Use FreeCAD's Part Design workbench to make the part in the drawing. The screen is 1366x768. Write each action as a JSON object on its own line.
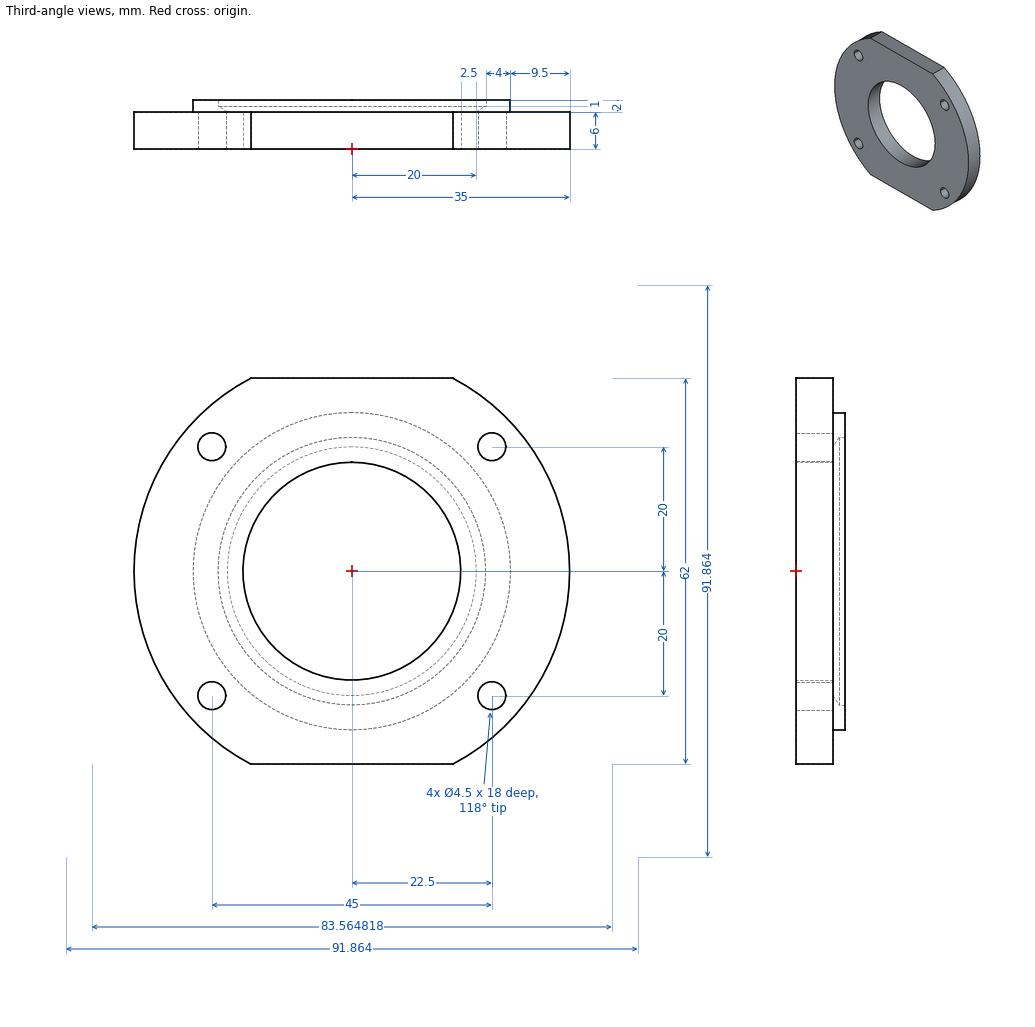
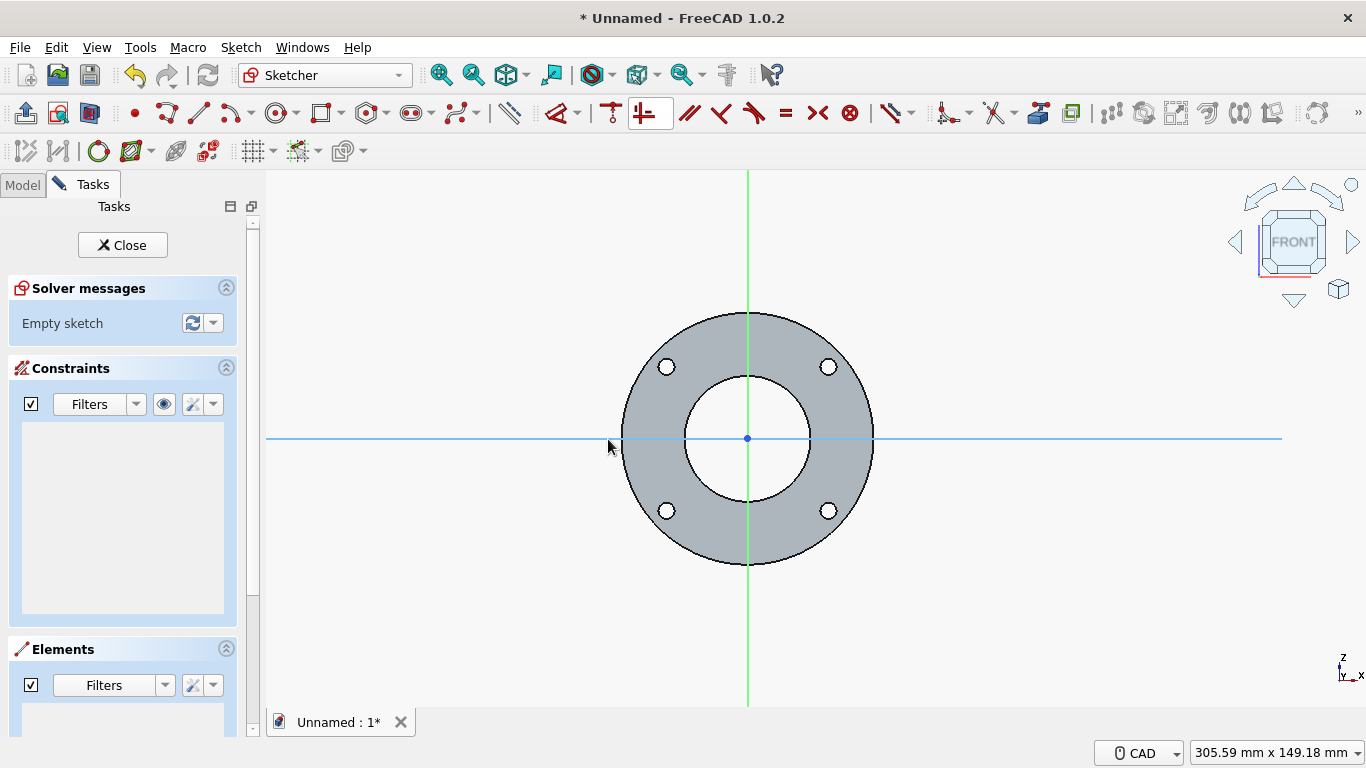
{"action": "left_click", "coordinate": [344, 114]}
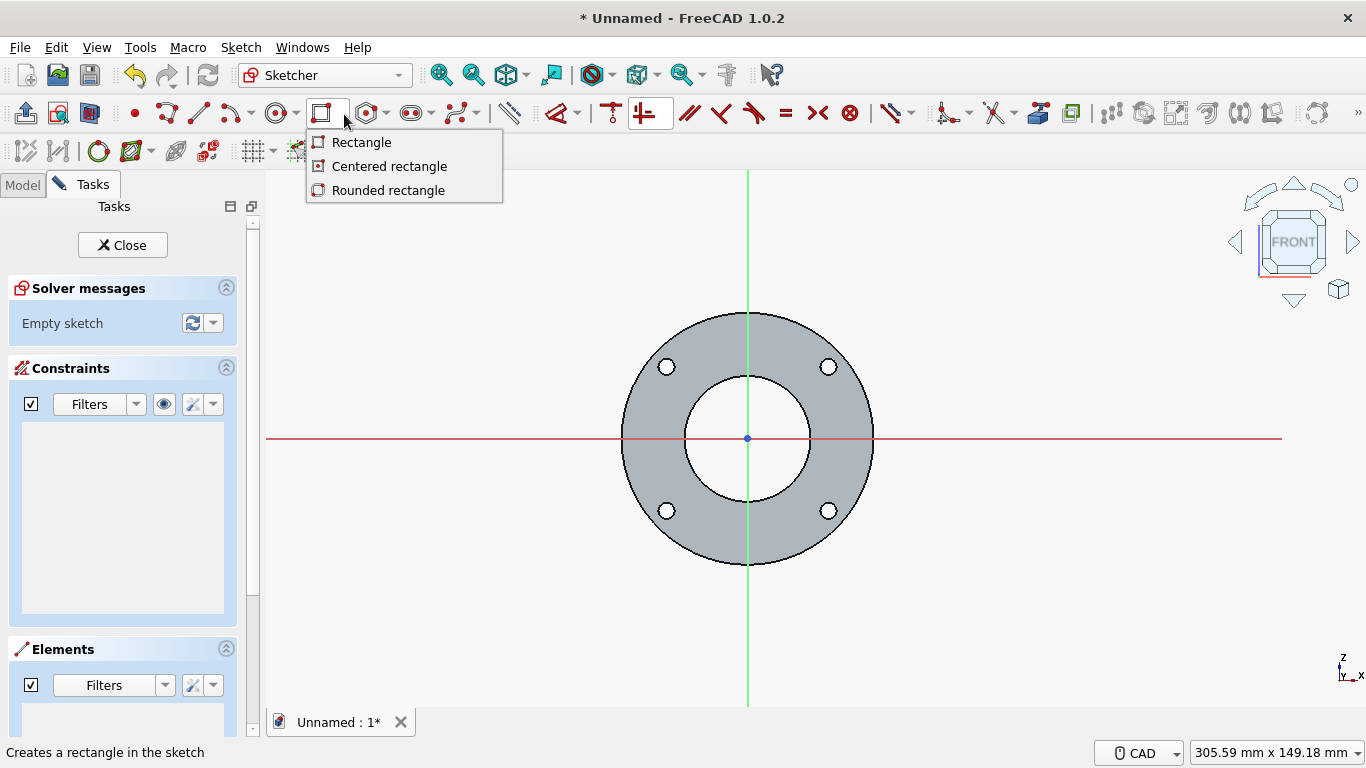
{"action": "left_click", "coordinate": [404, 166]}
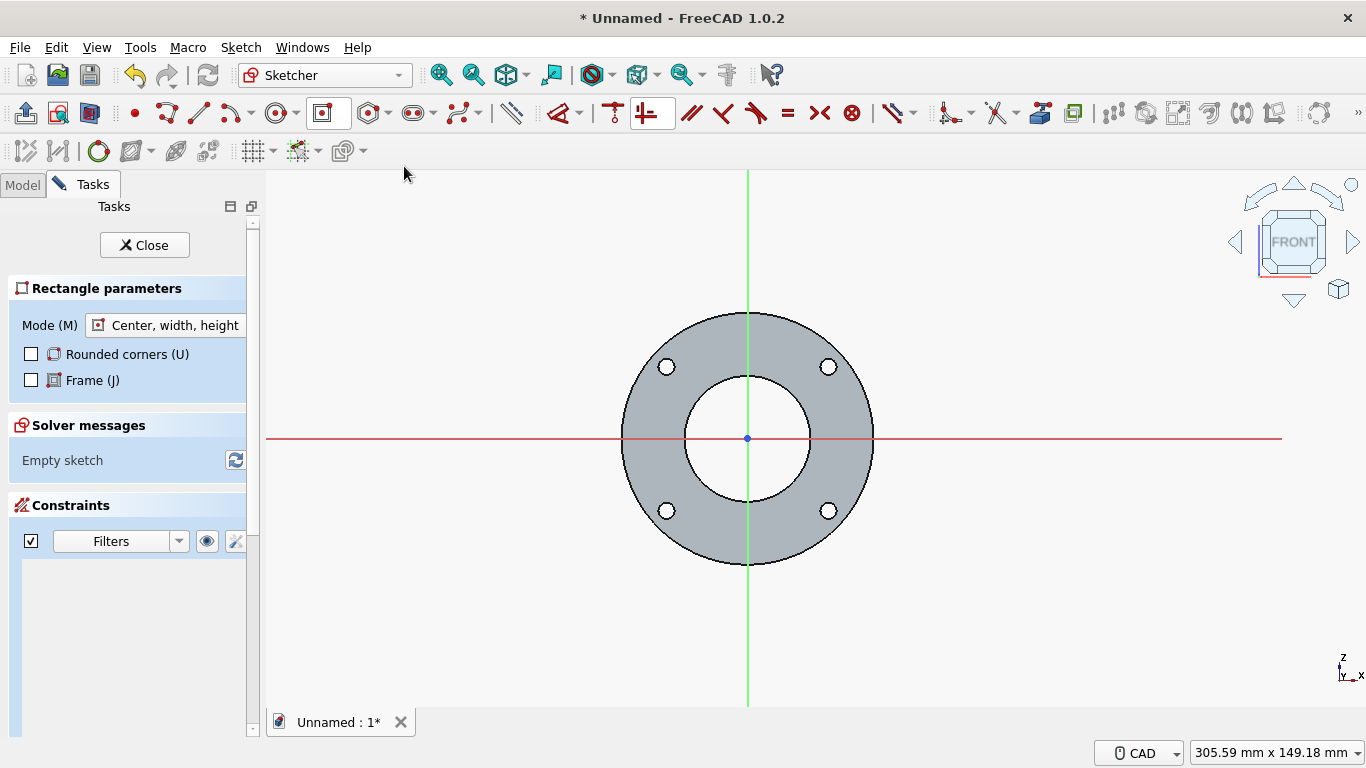
{"action": "left_click", "coordinate": [748, 439]}
{"action": "left_click", "coordinate": [913, 273]}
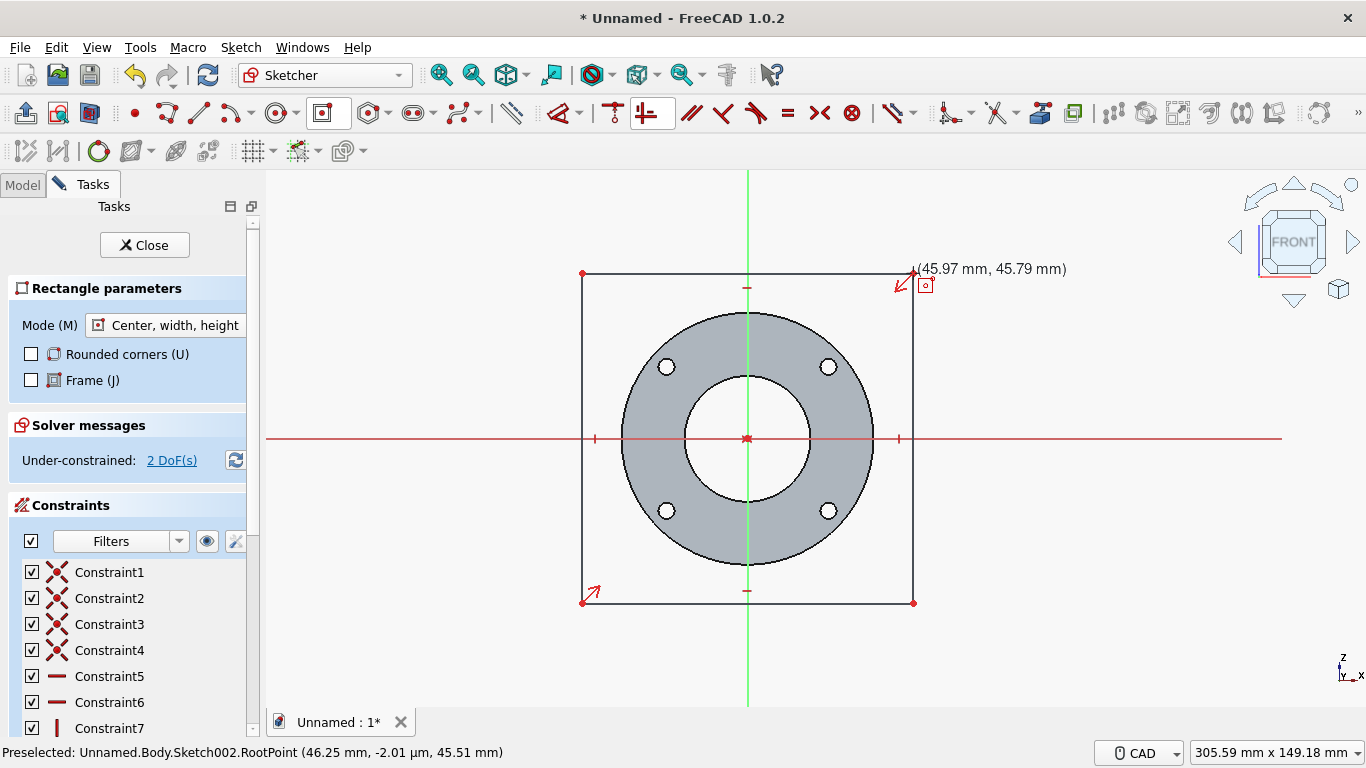
{"action": "left_click", "coordinate": [748, 439]}
{"action": "left_click", "coordinate": [898, 327]}
{"action": "key", "text": "Escape"}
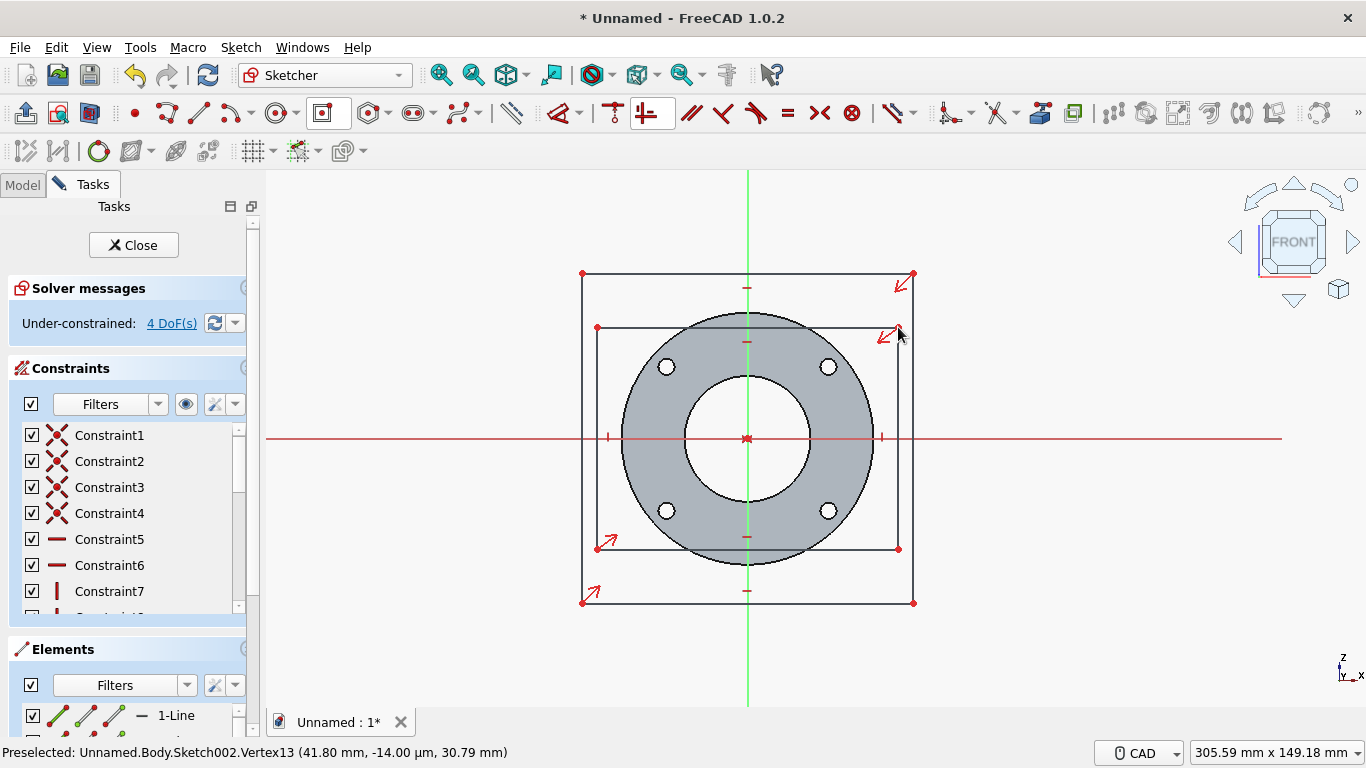
{"action": "left_click", "coordinate": [558, 114]}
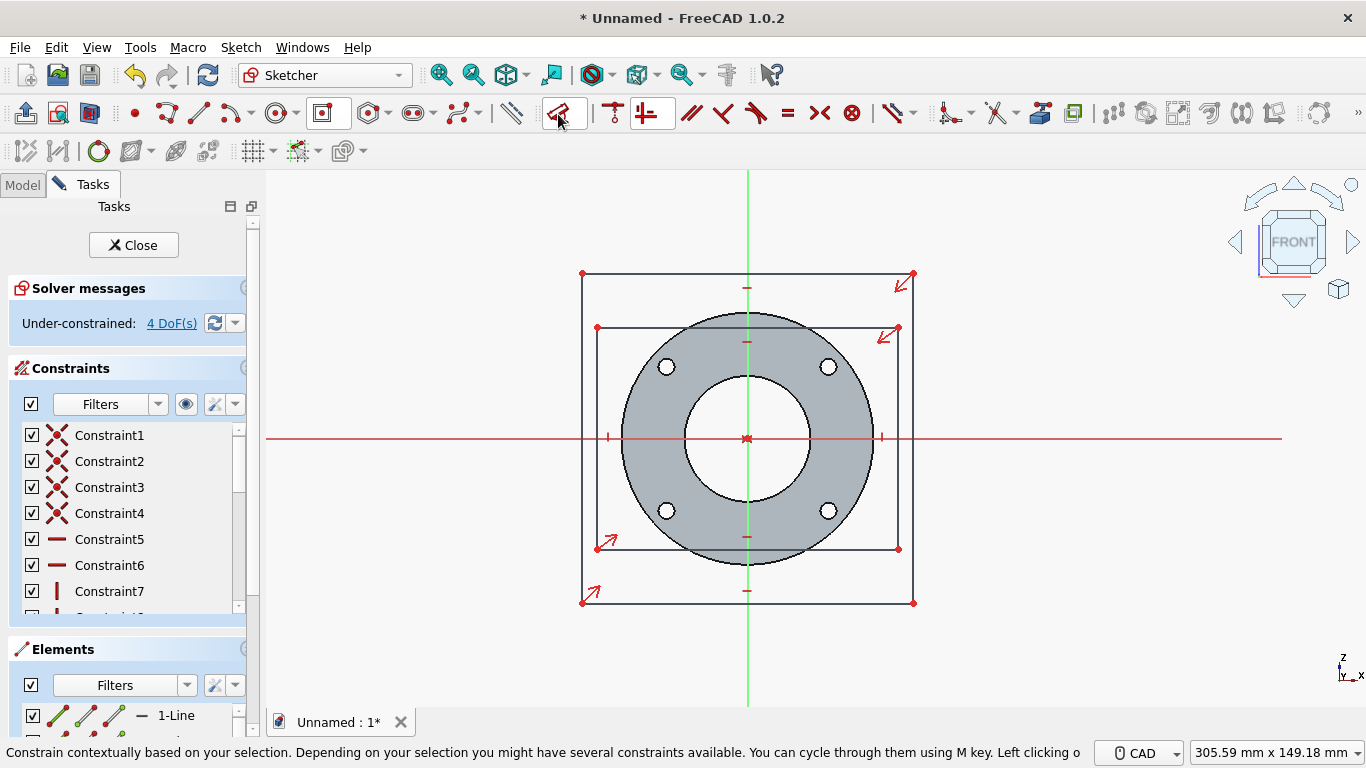
{"action": "left_click", "coordinate": [898, 483]}
{"action": "left_click", "coordinate": [932, 388]}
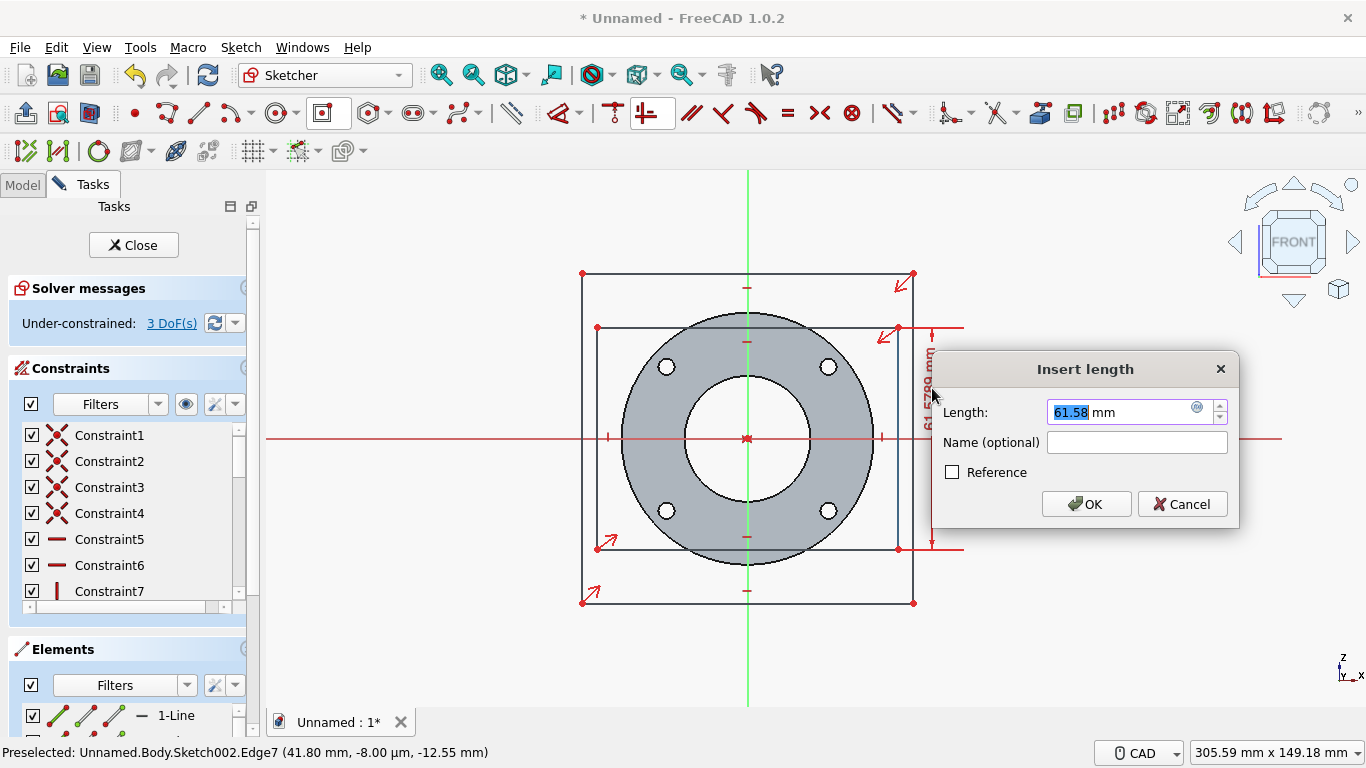
{"action": "type", "text": "62"}
{"action": "key", "text": "Return"}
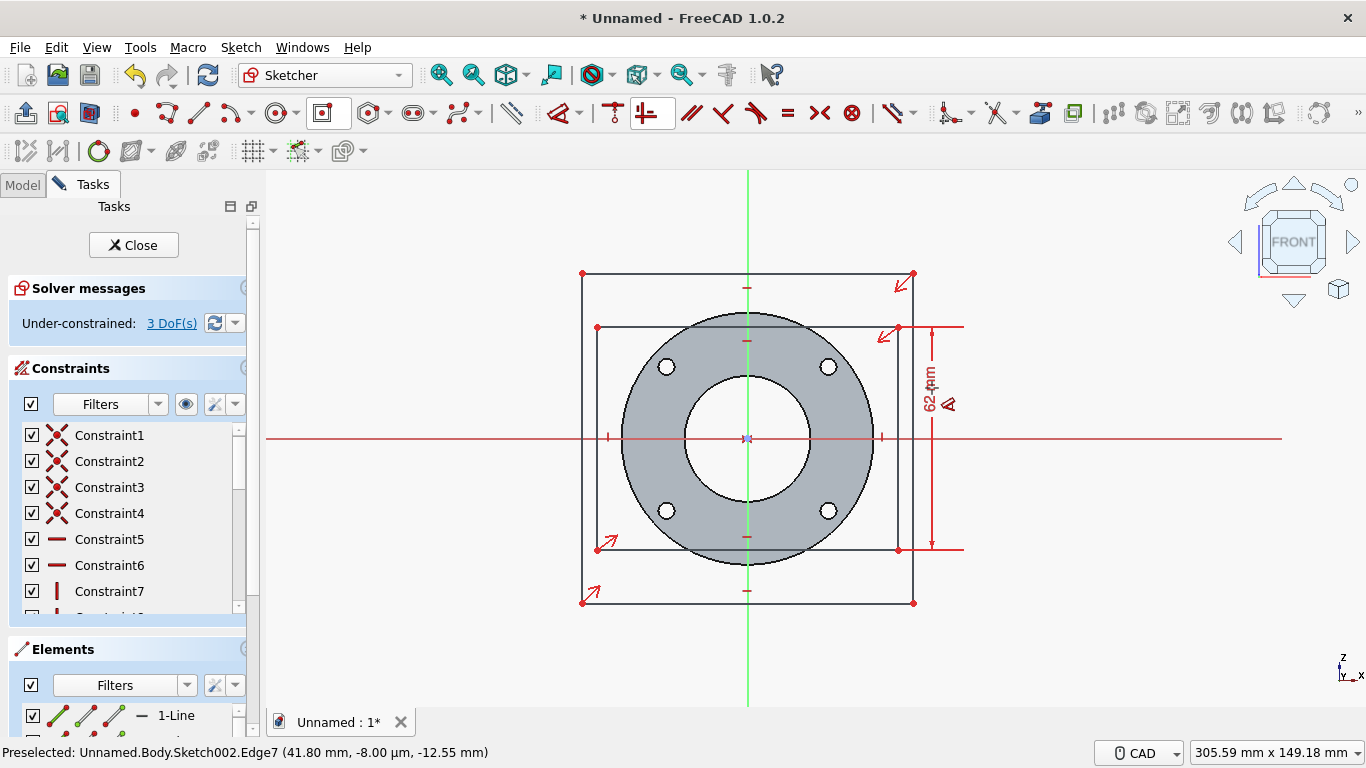
{"action": "left_click", "coordinate": [681, 604]}
{"action": "left_click", "coordinate": [671, 638]}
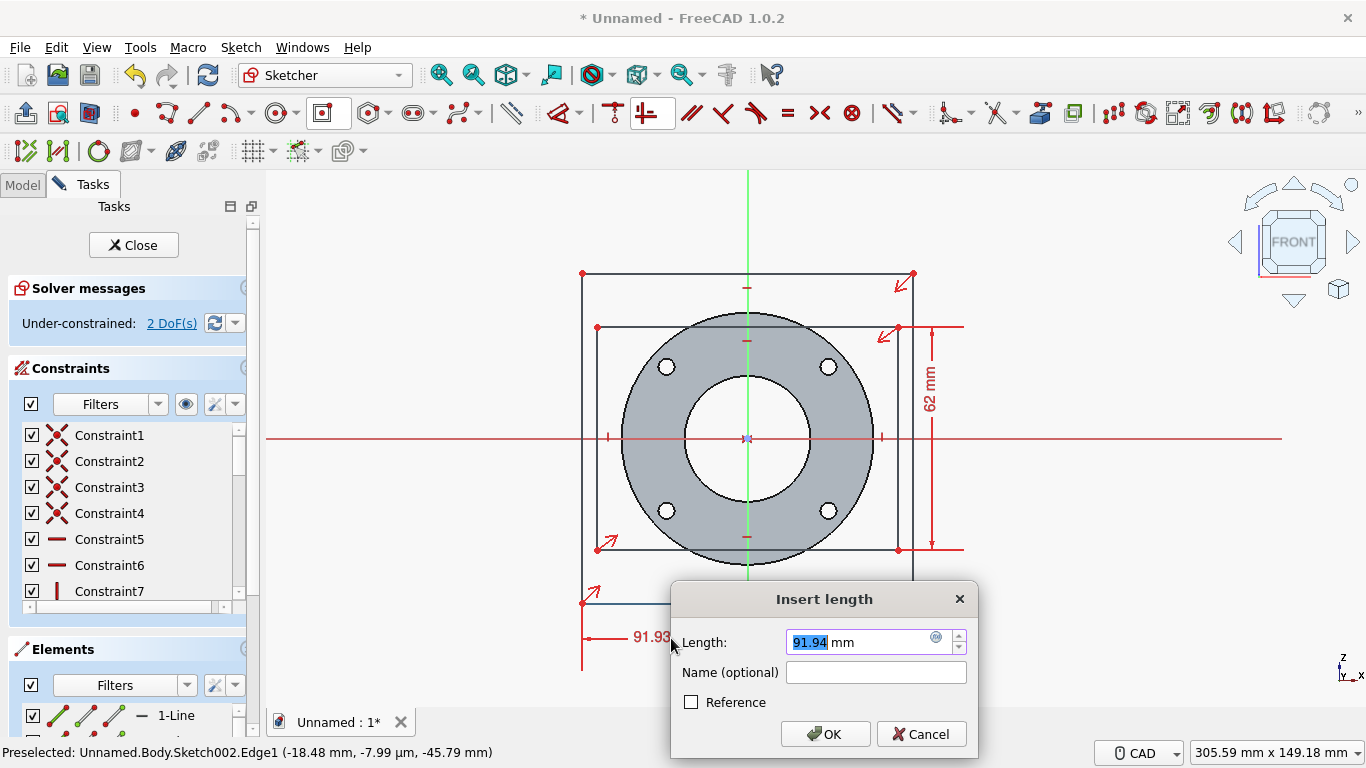
{"action": "type", "text": "91.864"}
{"action": "key", "text": "Return"}